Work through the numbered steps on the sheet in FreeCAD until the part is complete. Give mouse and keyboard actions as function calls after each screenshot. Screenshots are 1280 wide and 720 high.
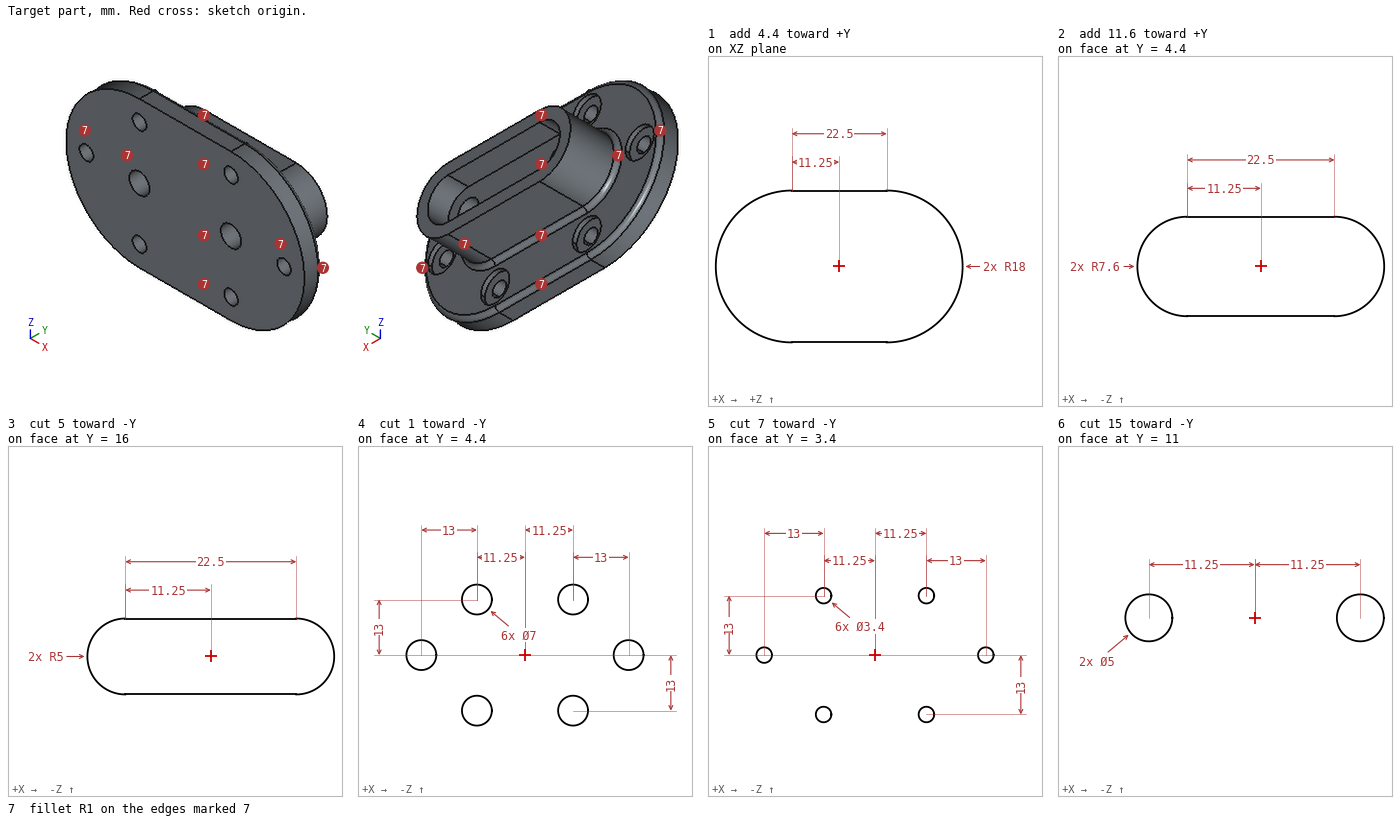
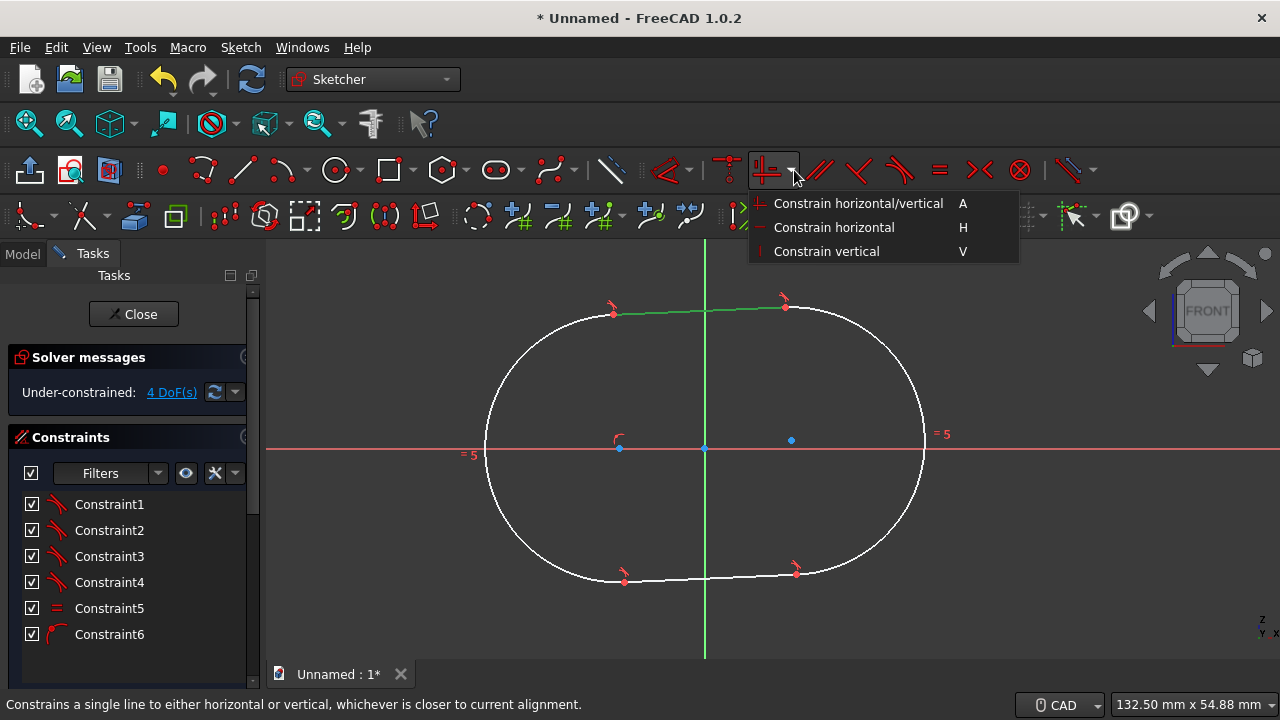
click(884, 227)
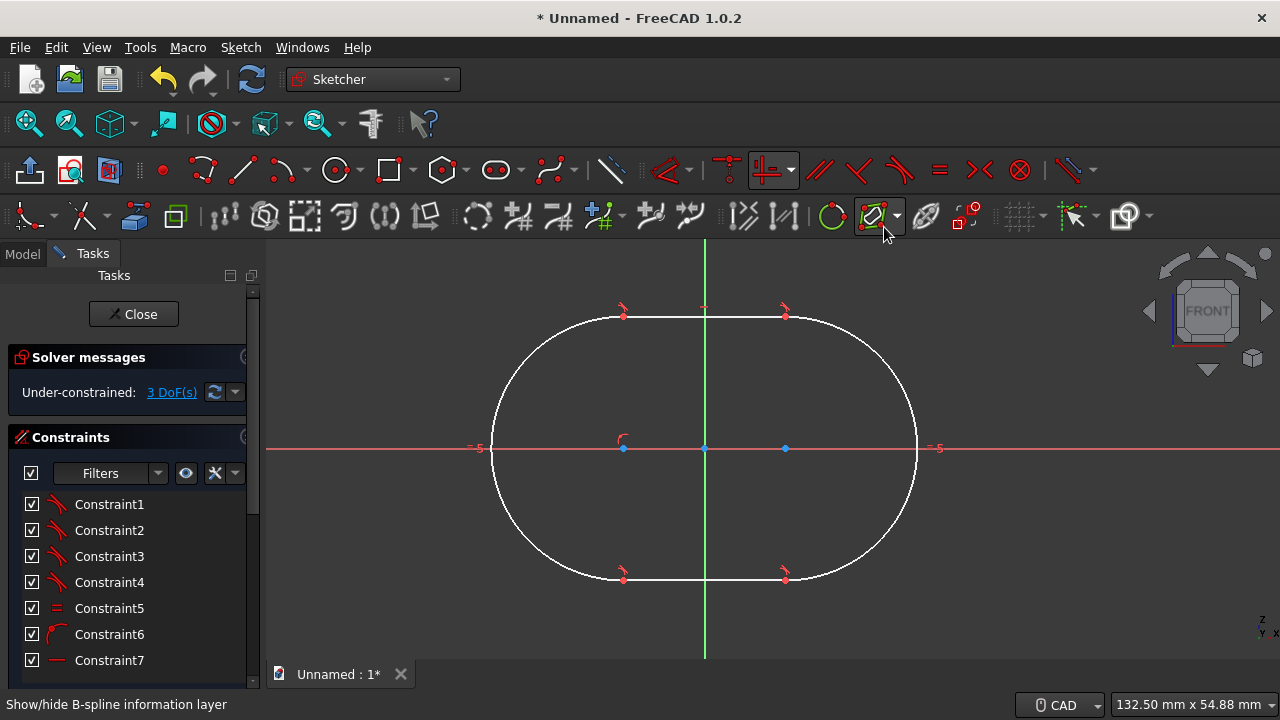
click(666, 170)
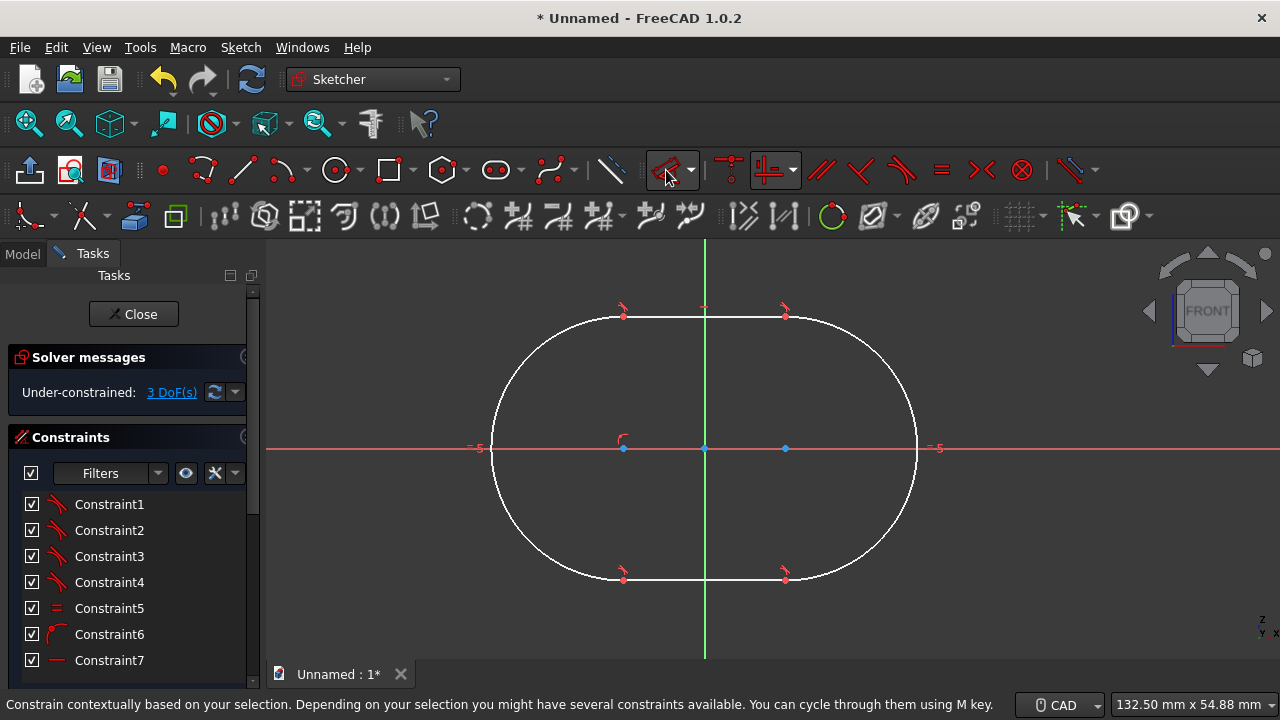
click(517, 371)
click(491, 352)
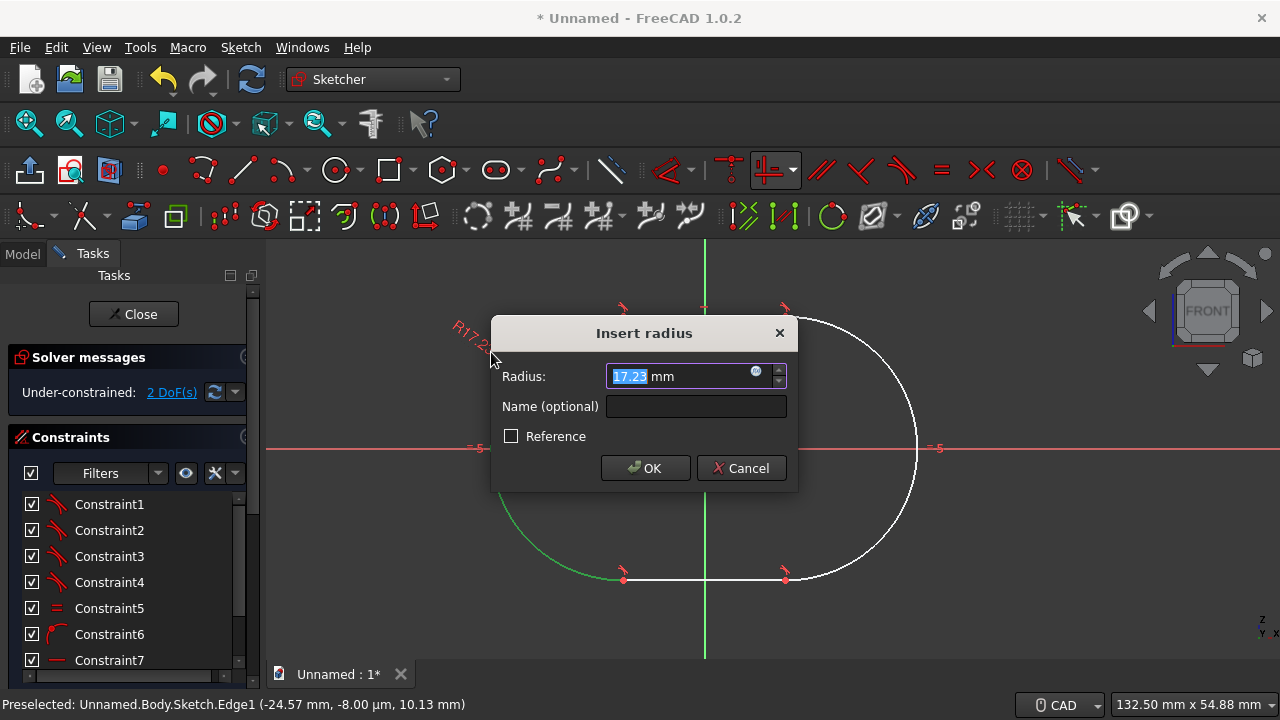
text(18)
key(Return)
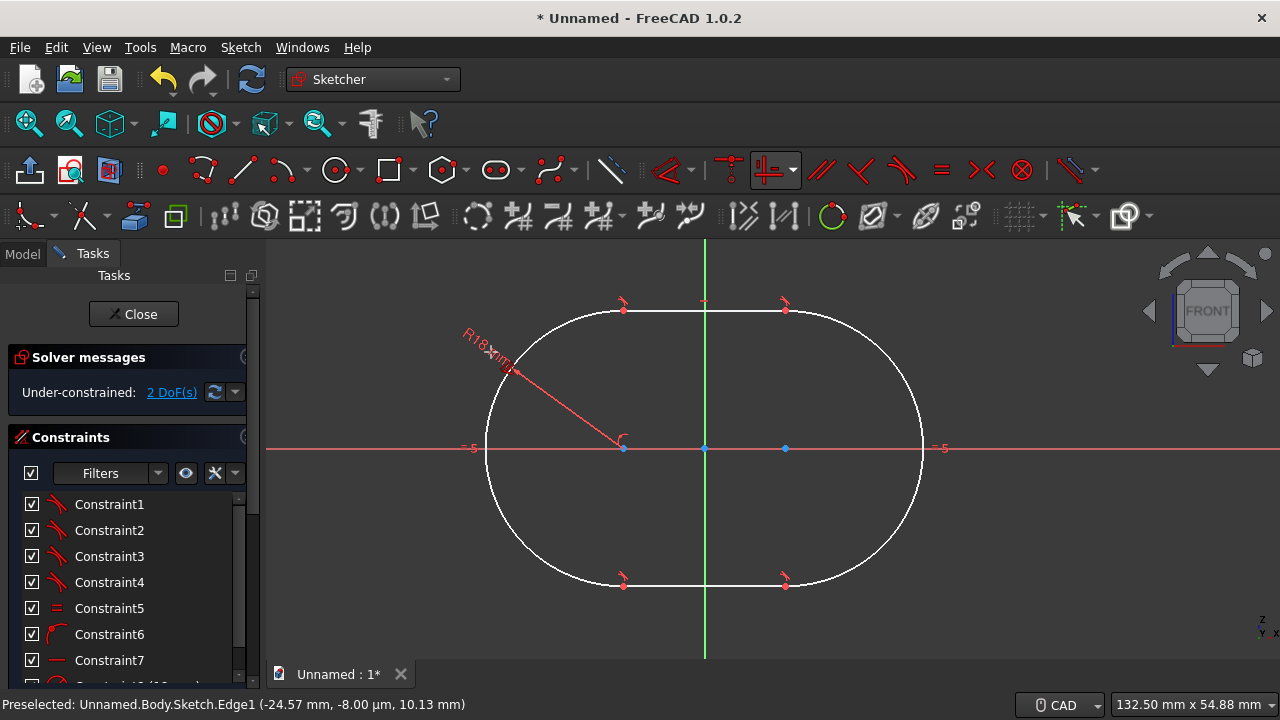
click(672, 311)
click(667, 277)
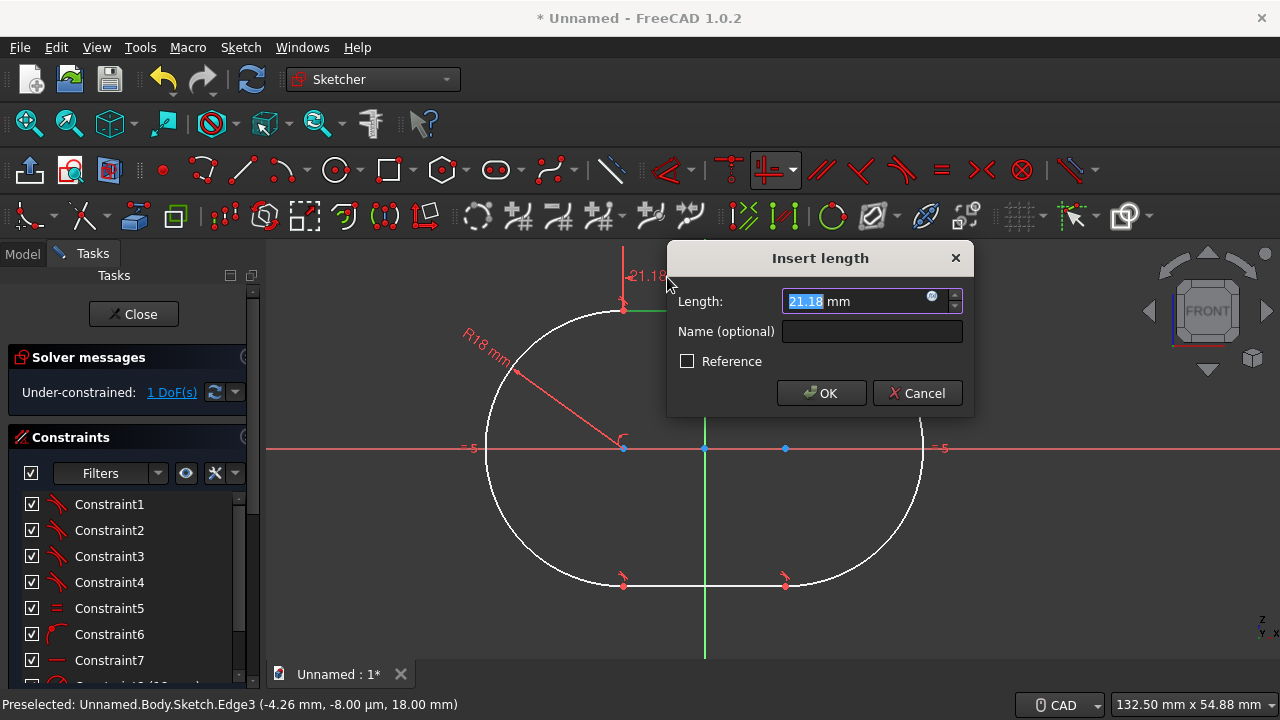
text(22.5)
key(Return)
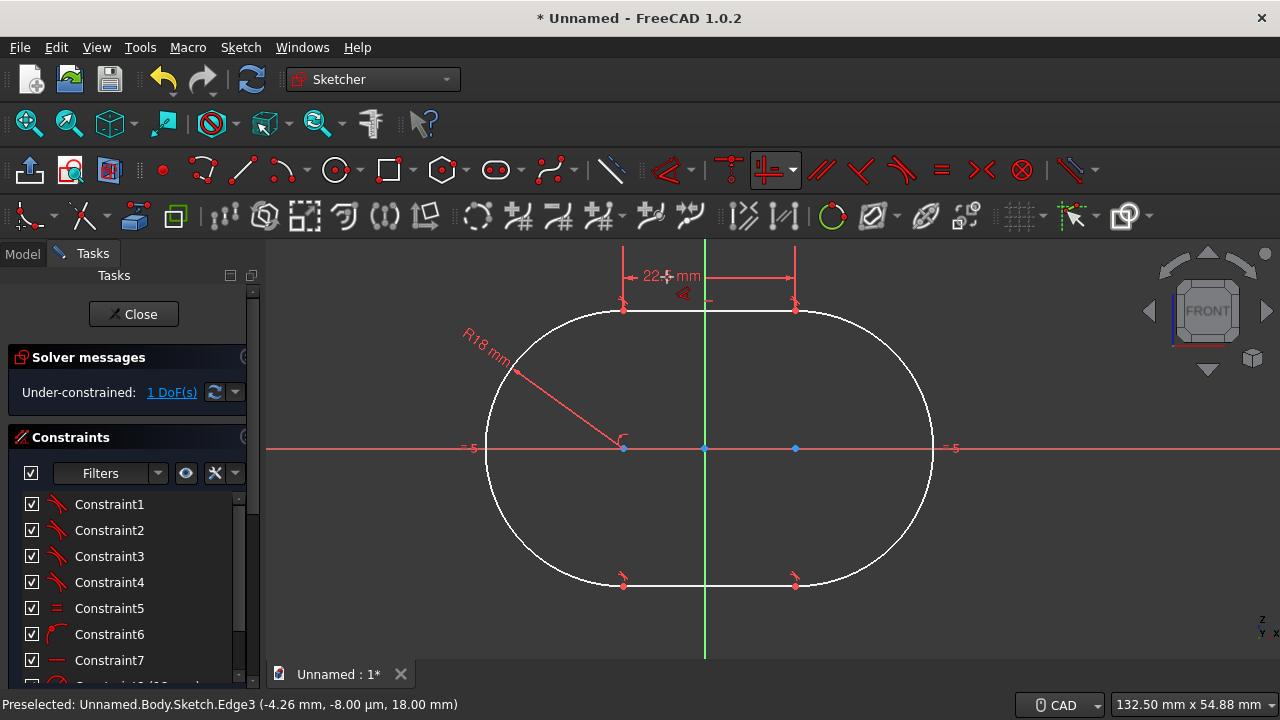
click(623, 311)
click(664, 483)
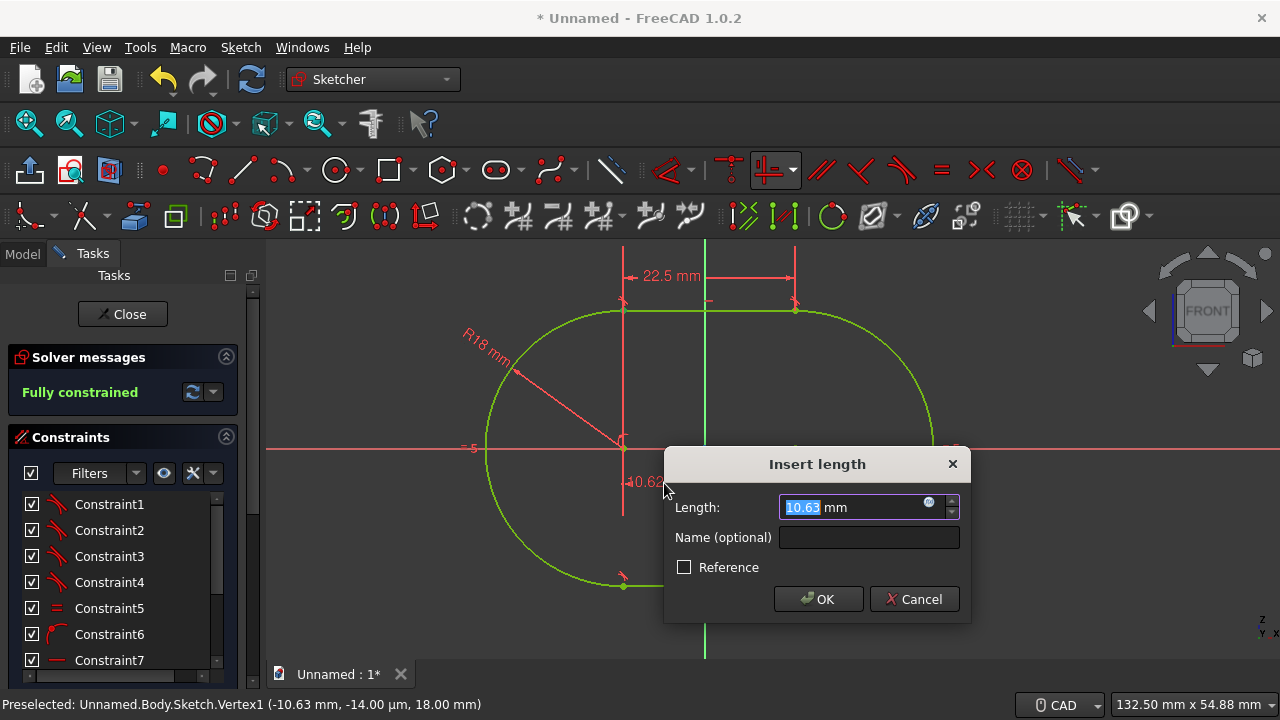
text(11.25)
key(Return)
key(Escape)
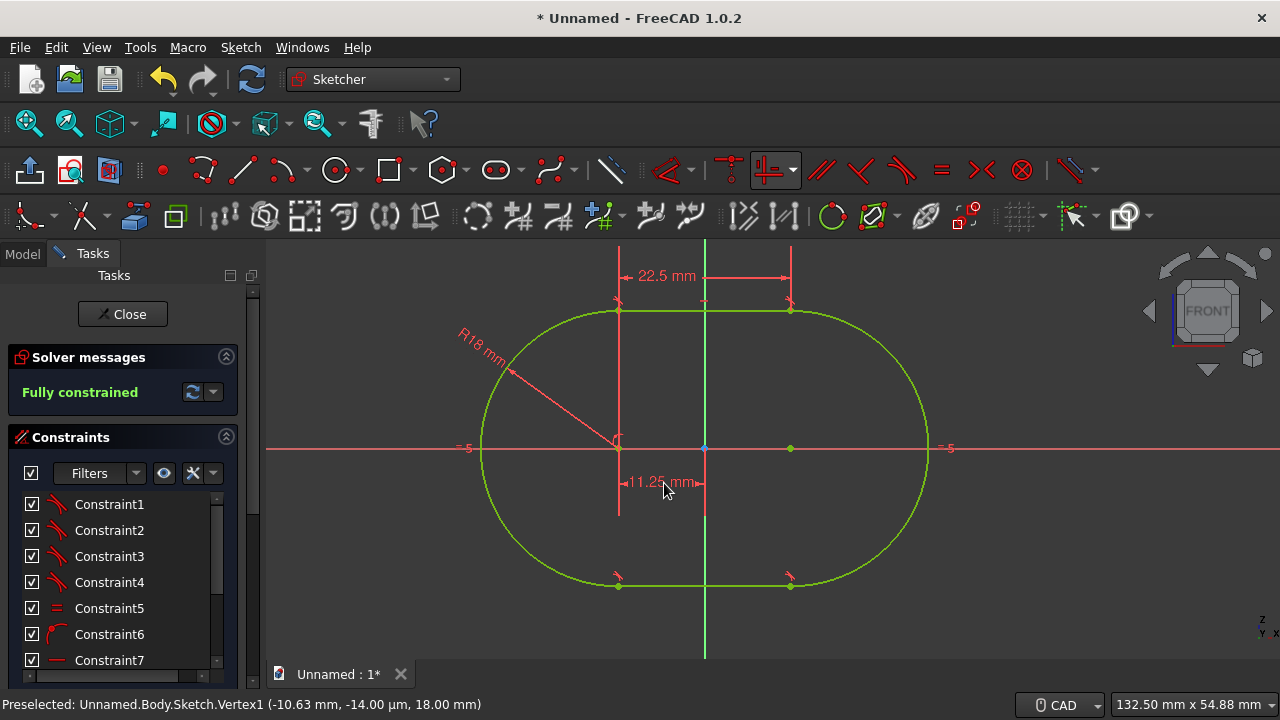
click(123, 314)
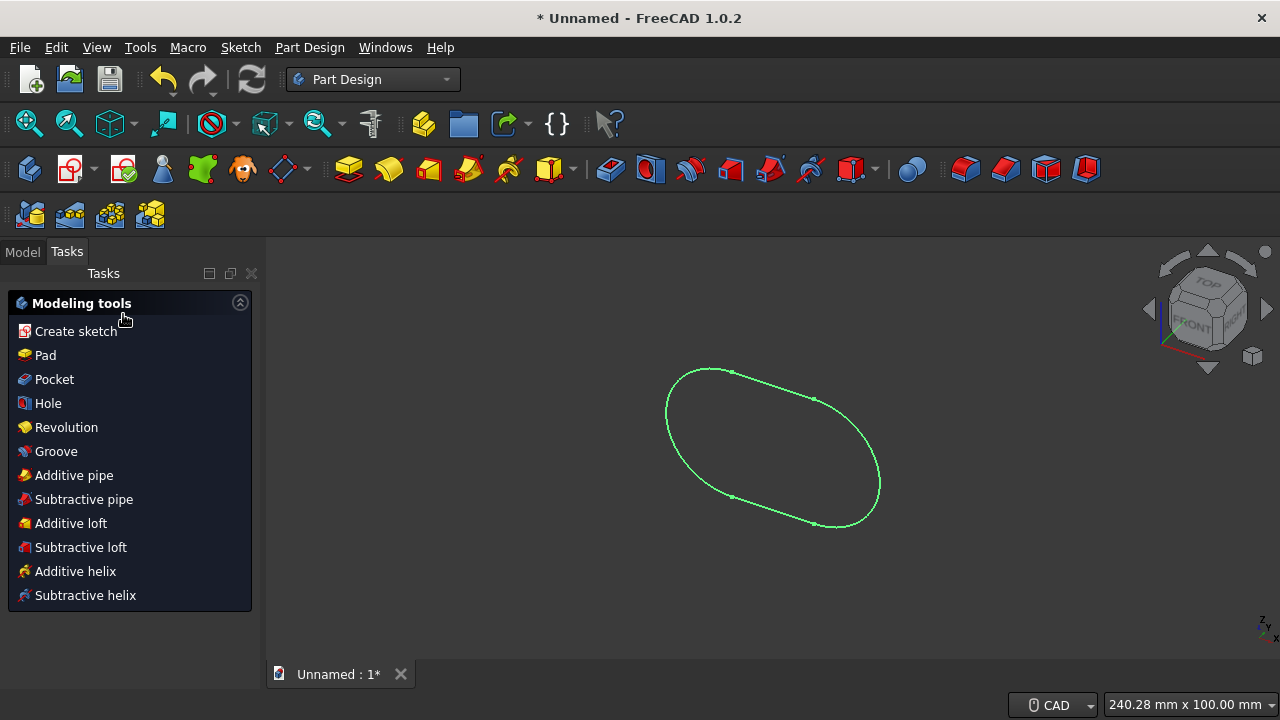
click(350, 170)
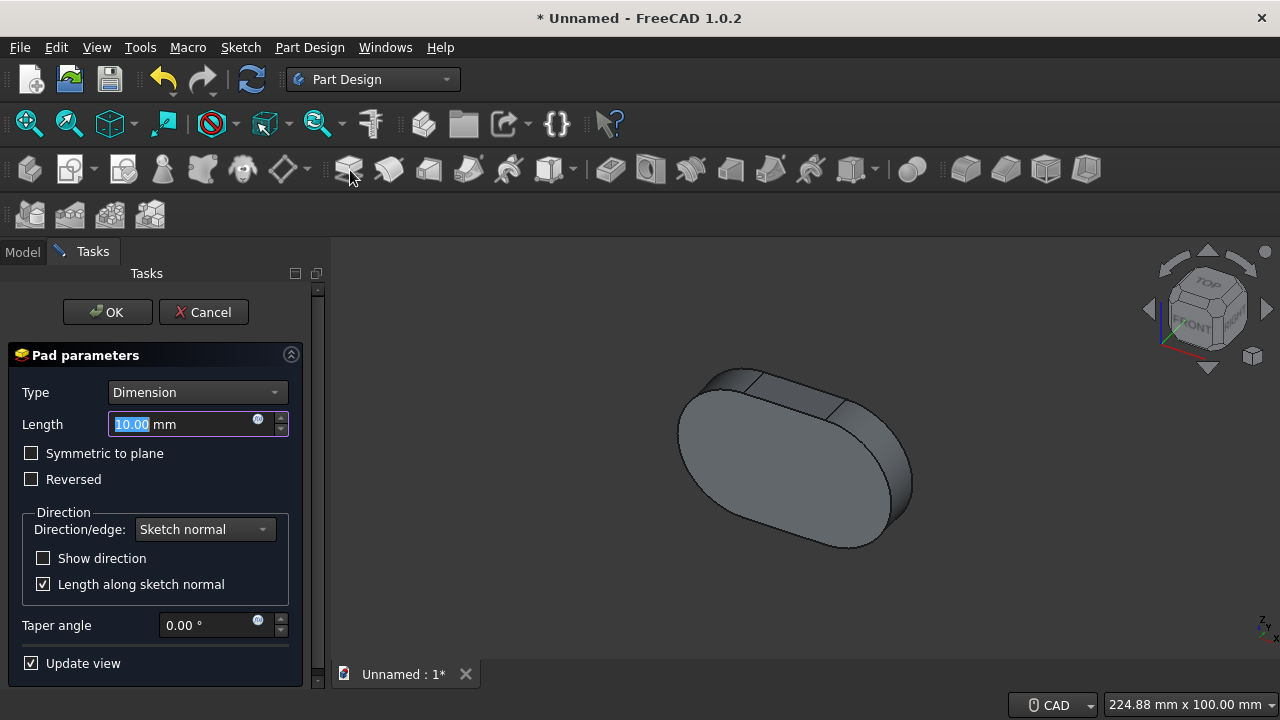
text(4.4)
key(Tab)